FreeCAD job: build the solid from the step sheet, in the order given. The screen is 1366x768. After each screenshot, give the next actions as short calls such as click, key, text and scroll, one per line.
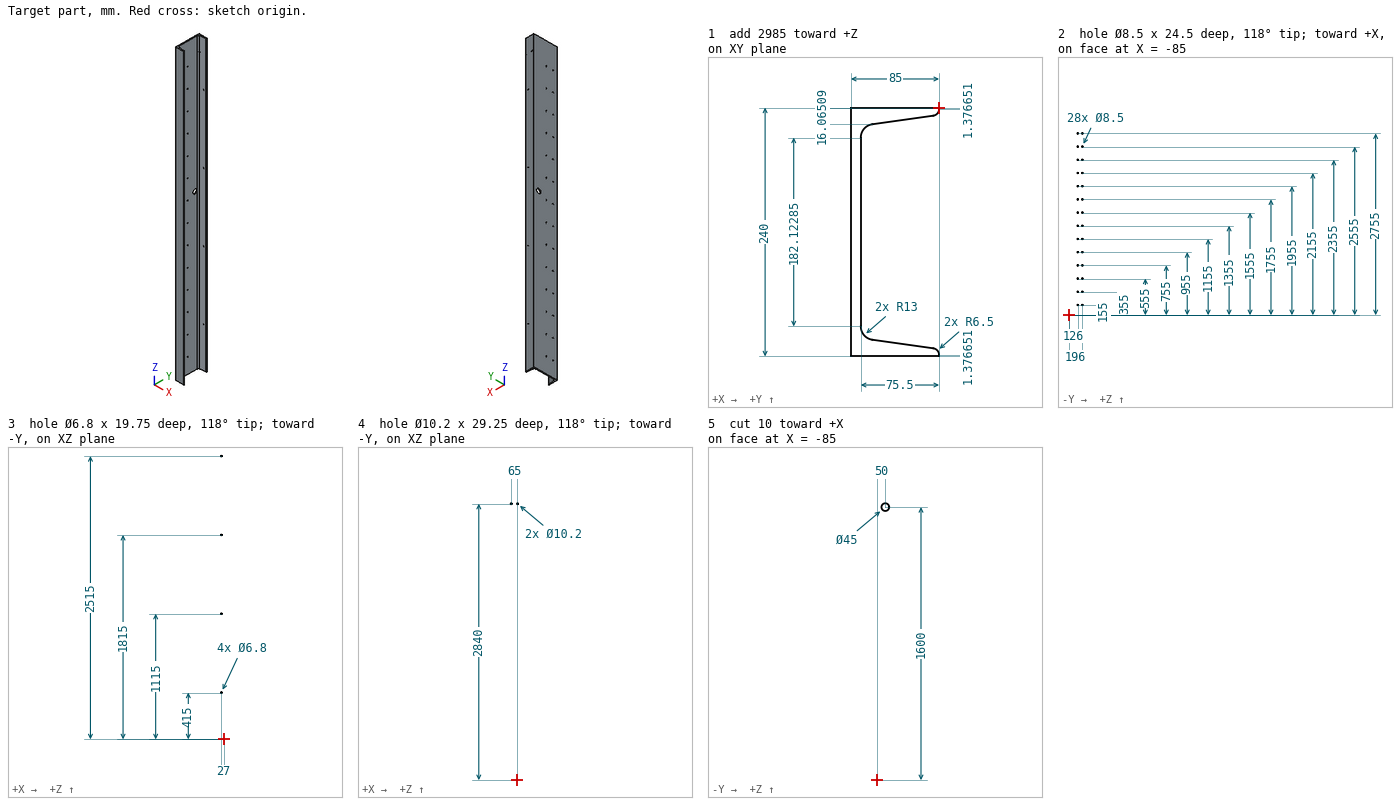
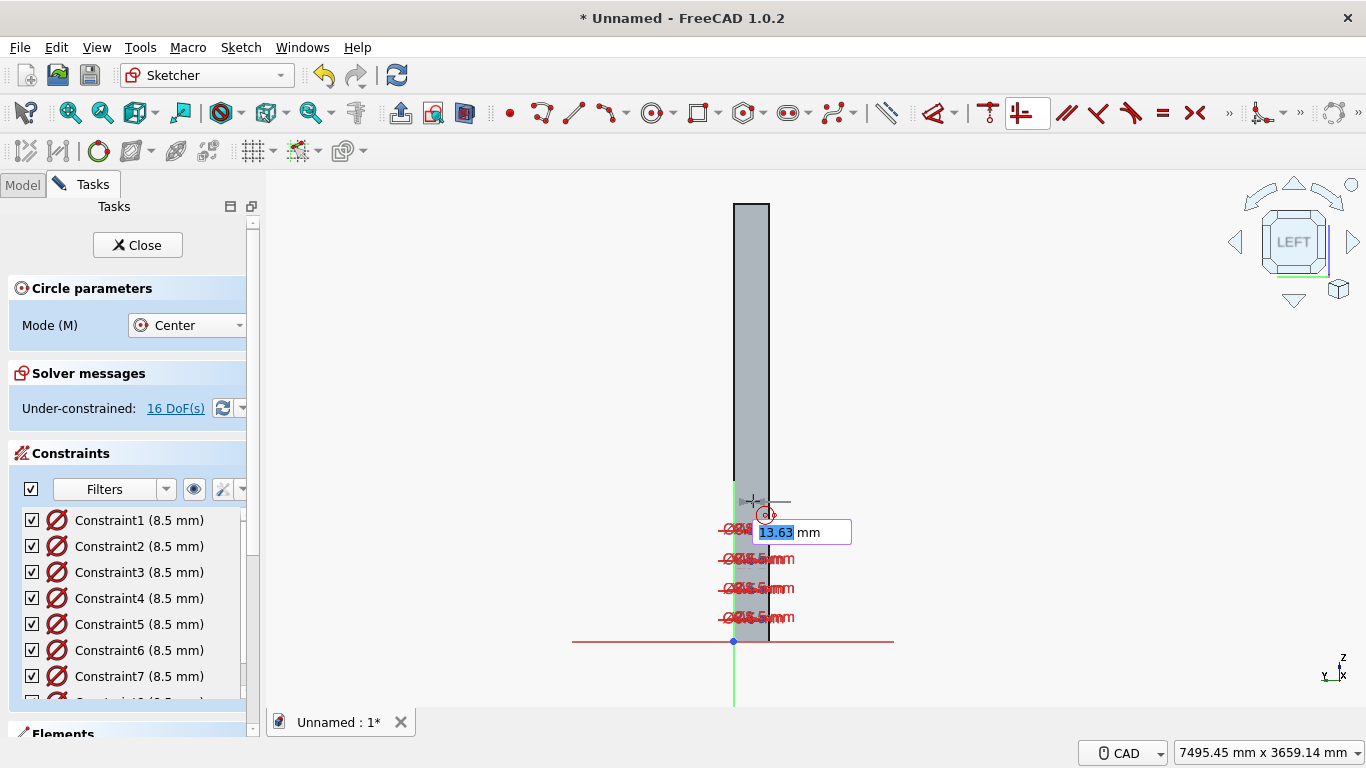
text(8.5)
key(Return)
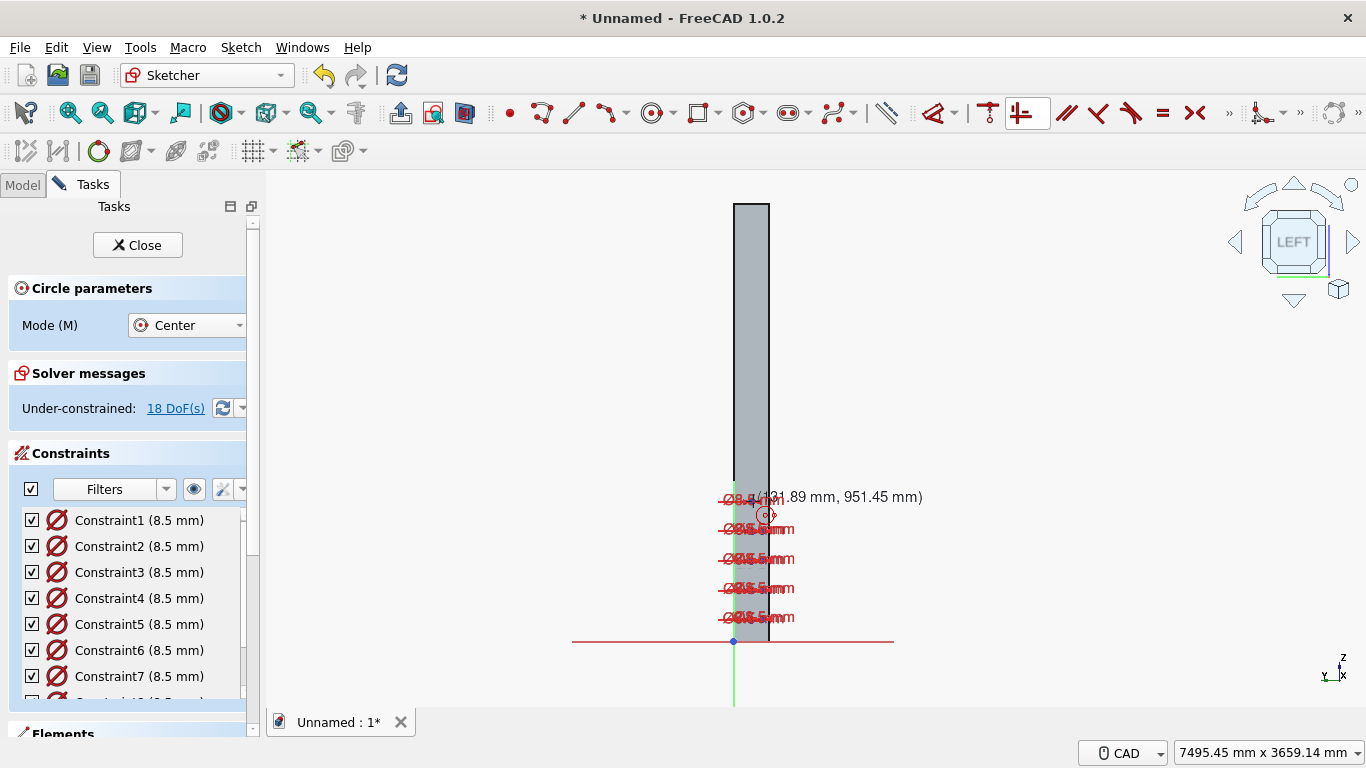
scroll(762, 501, up, 18)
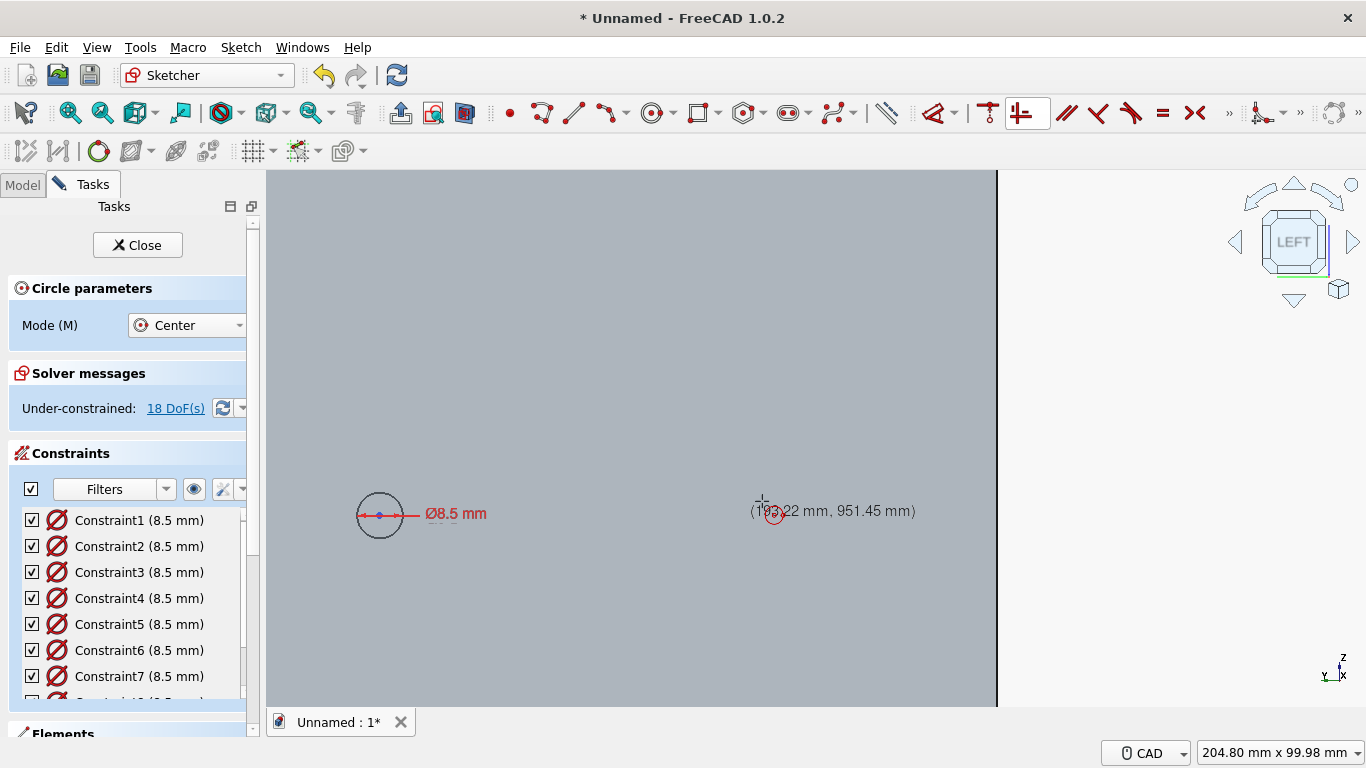
scroll(762, 501, down, 18)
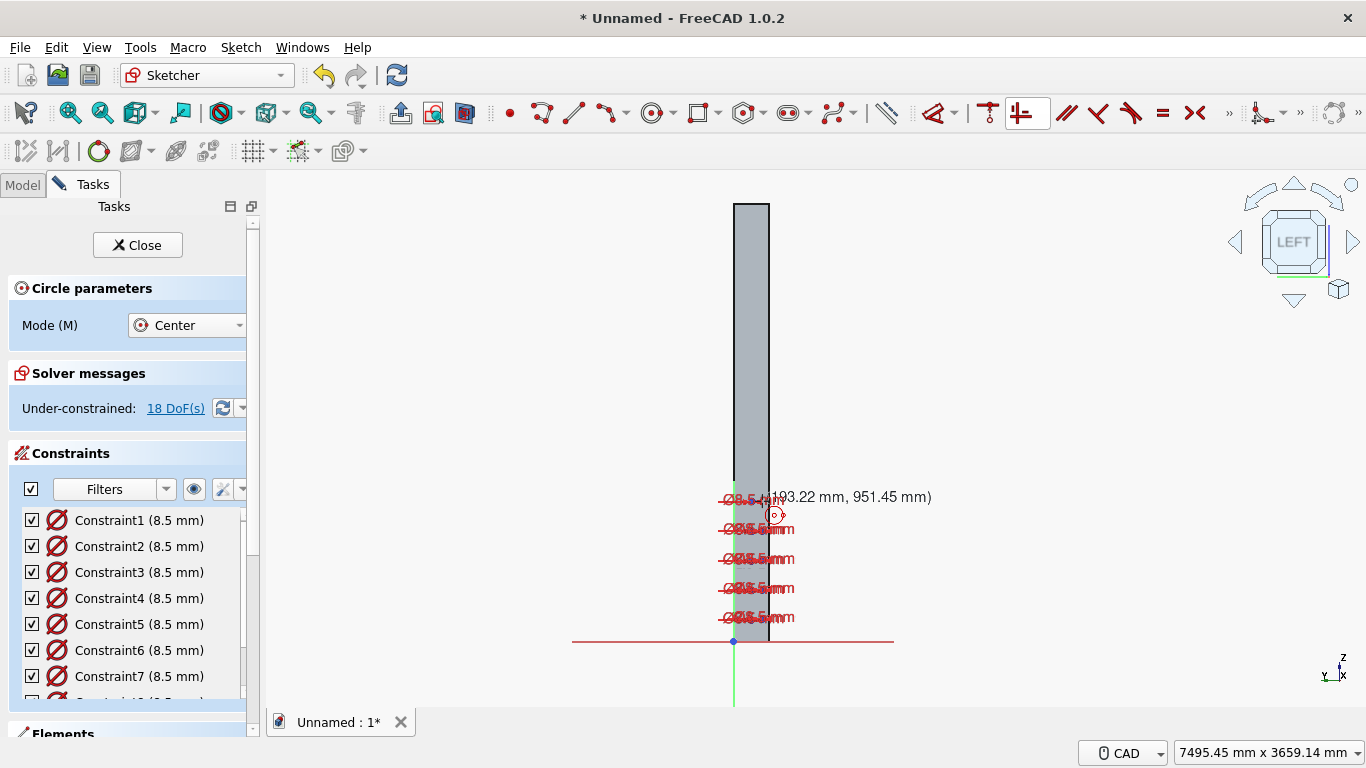
scroll(762, 501, up, 3)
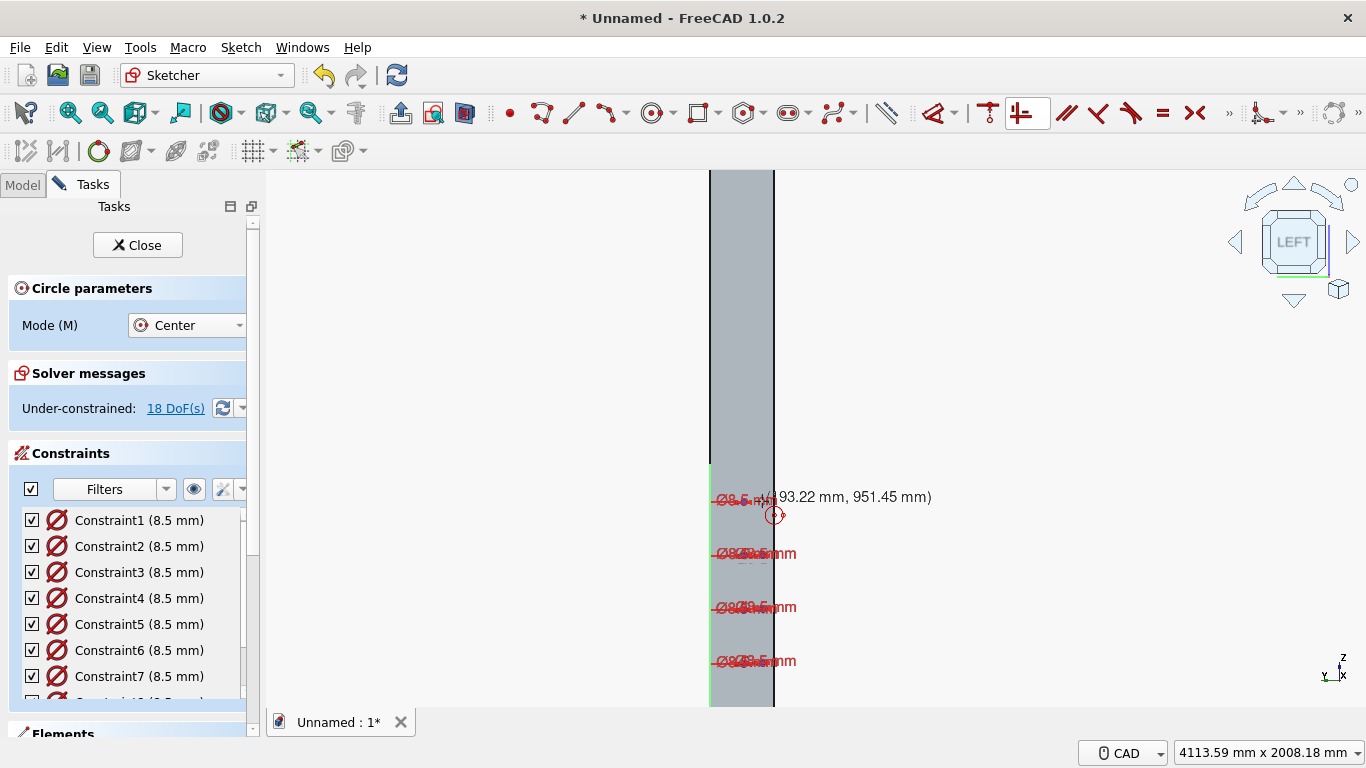
click(762, 501)
move(763, 501)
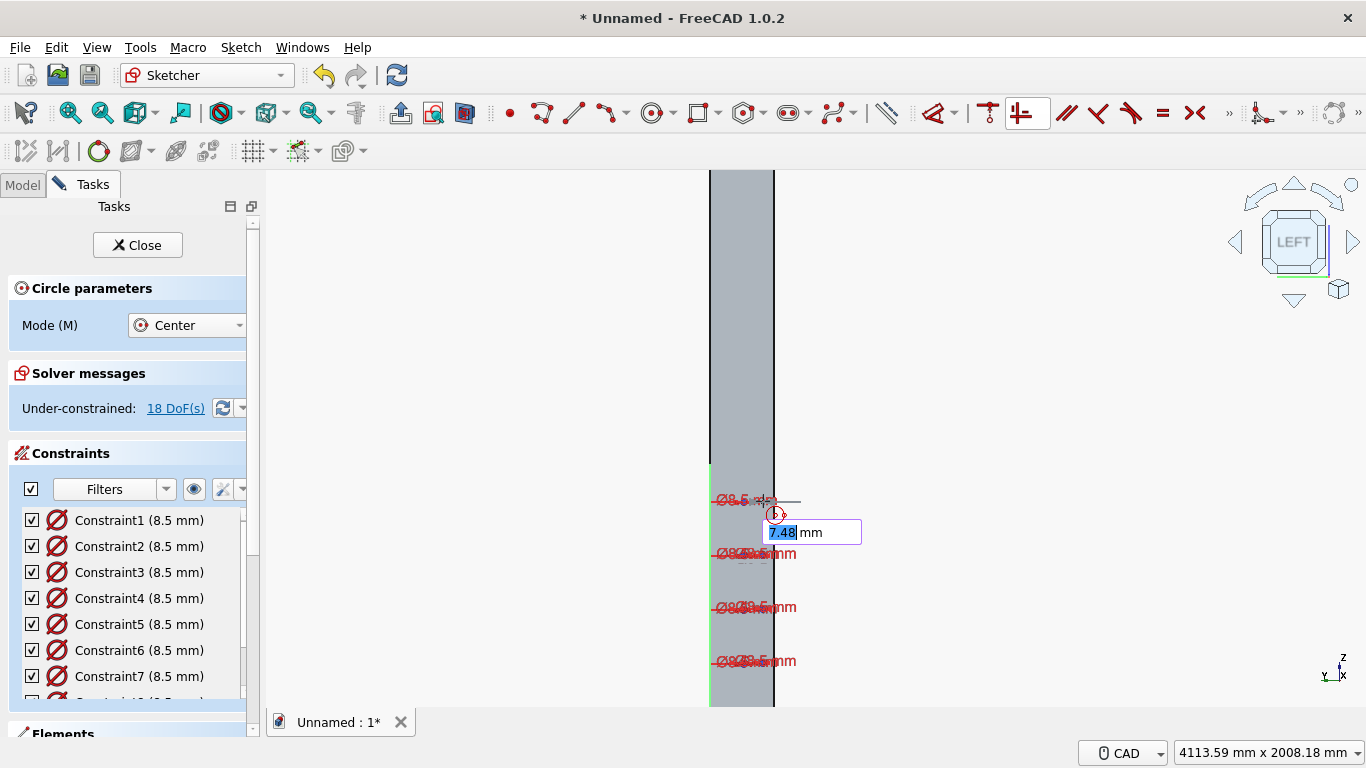
text(8.5)
key(Return)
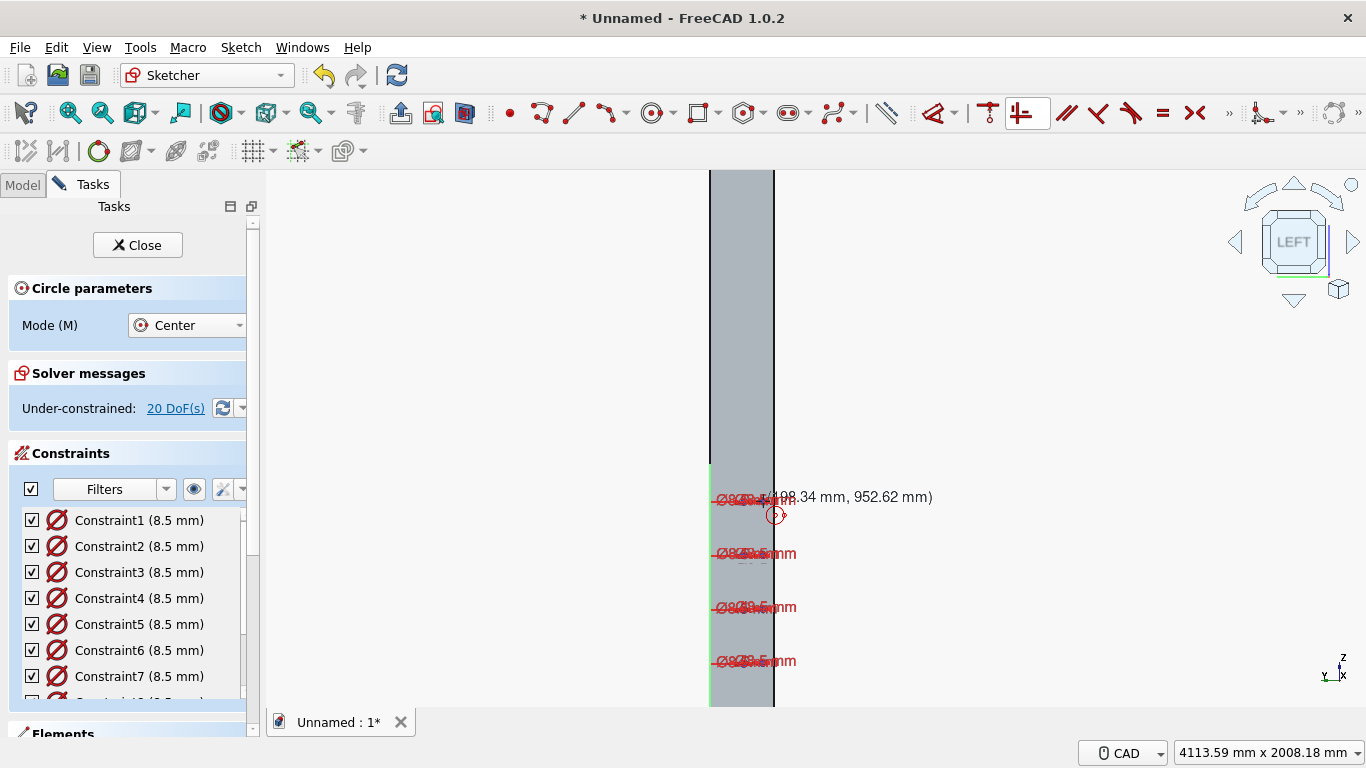
scroll(744, 448, up, 15)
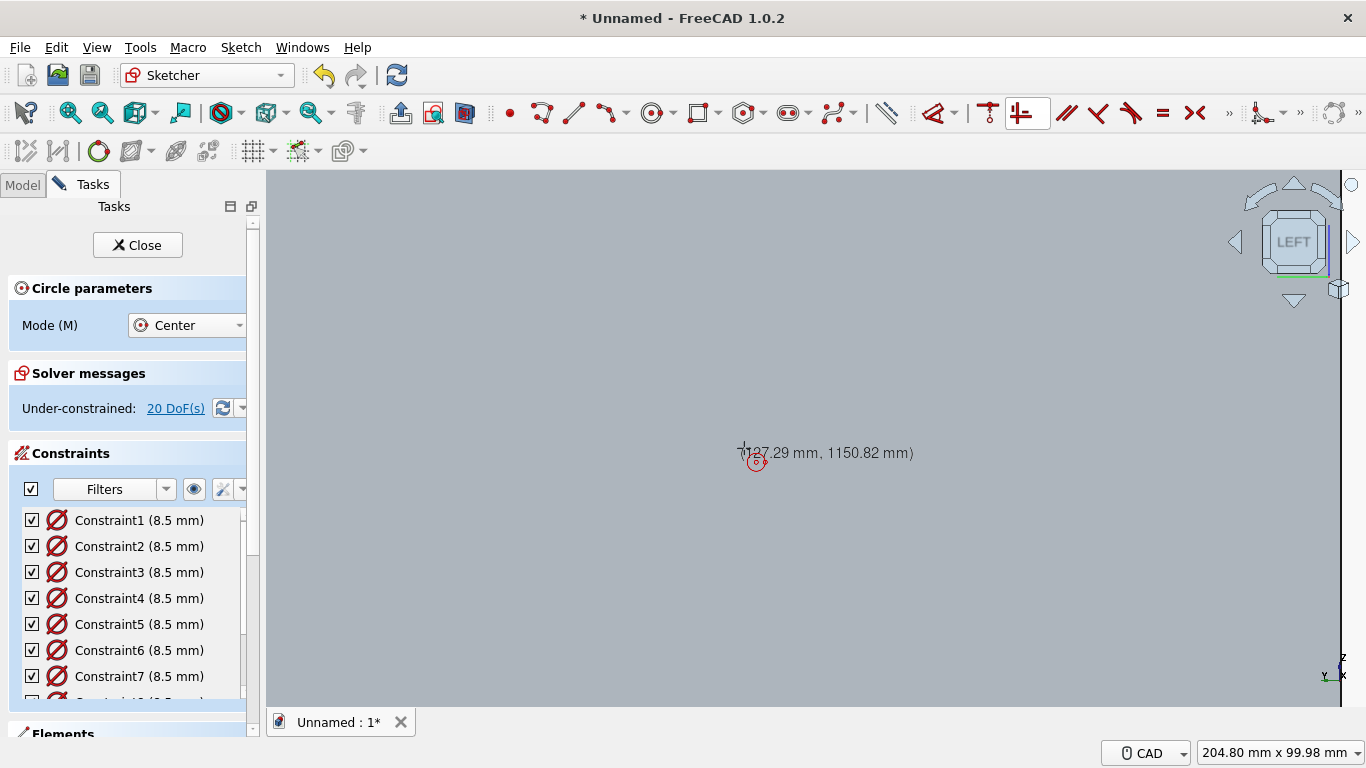
scroll(752, 472, down, 18)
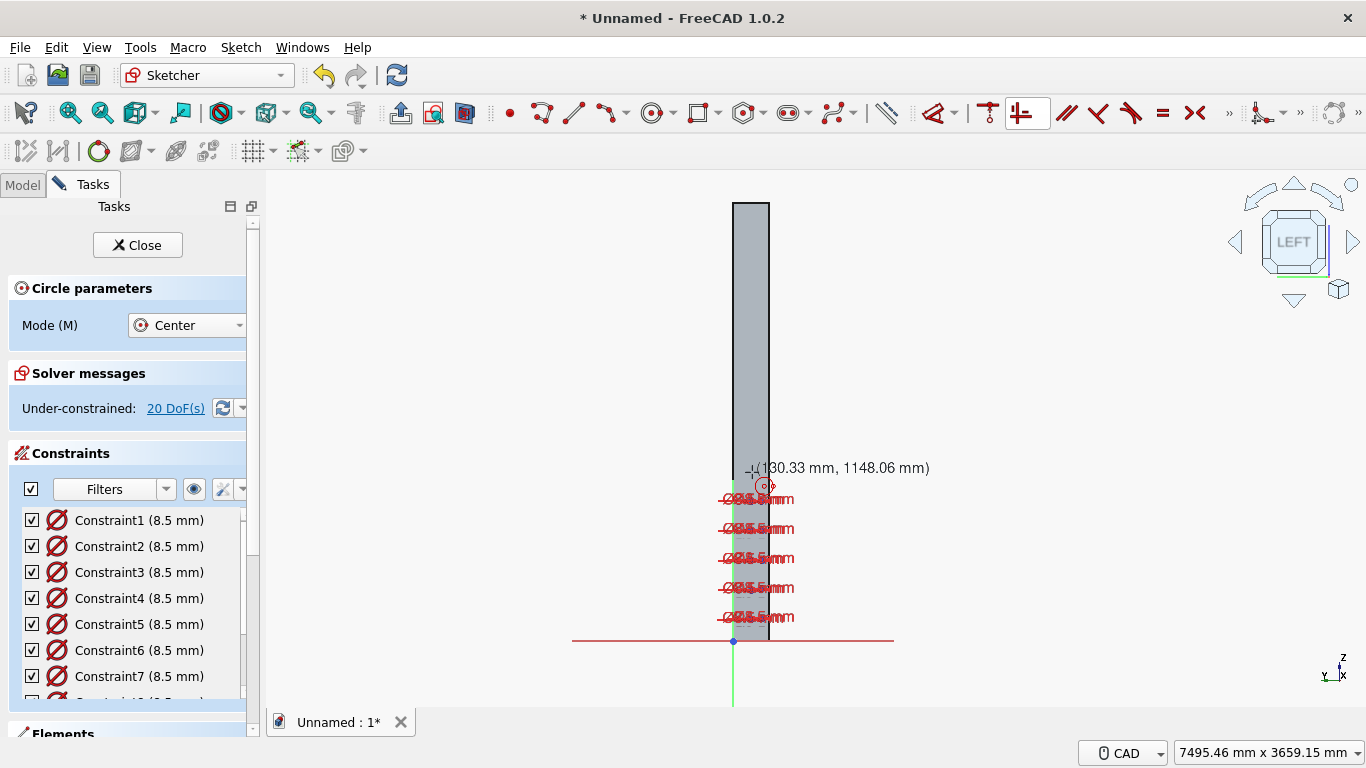
click(752, 472)
move(752, 471)